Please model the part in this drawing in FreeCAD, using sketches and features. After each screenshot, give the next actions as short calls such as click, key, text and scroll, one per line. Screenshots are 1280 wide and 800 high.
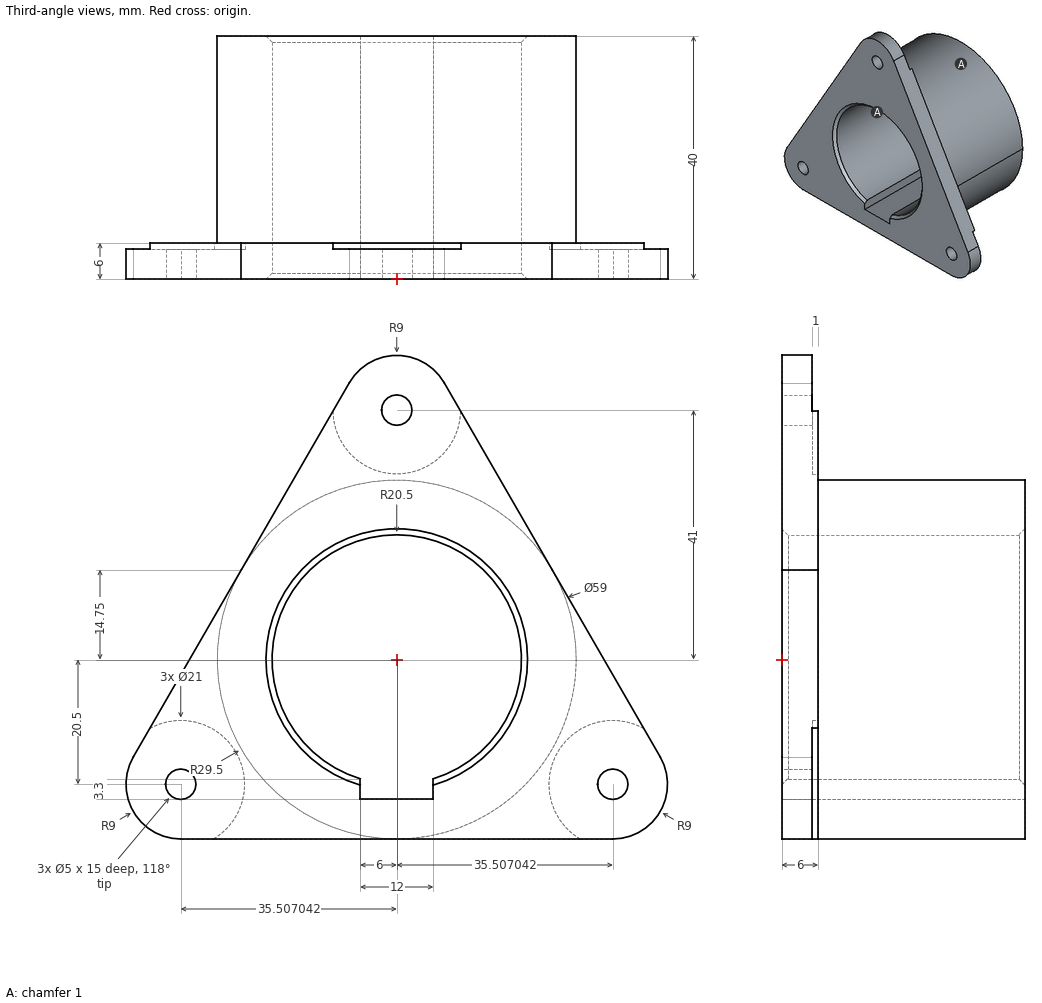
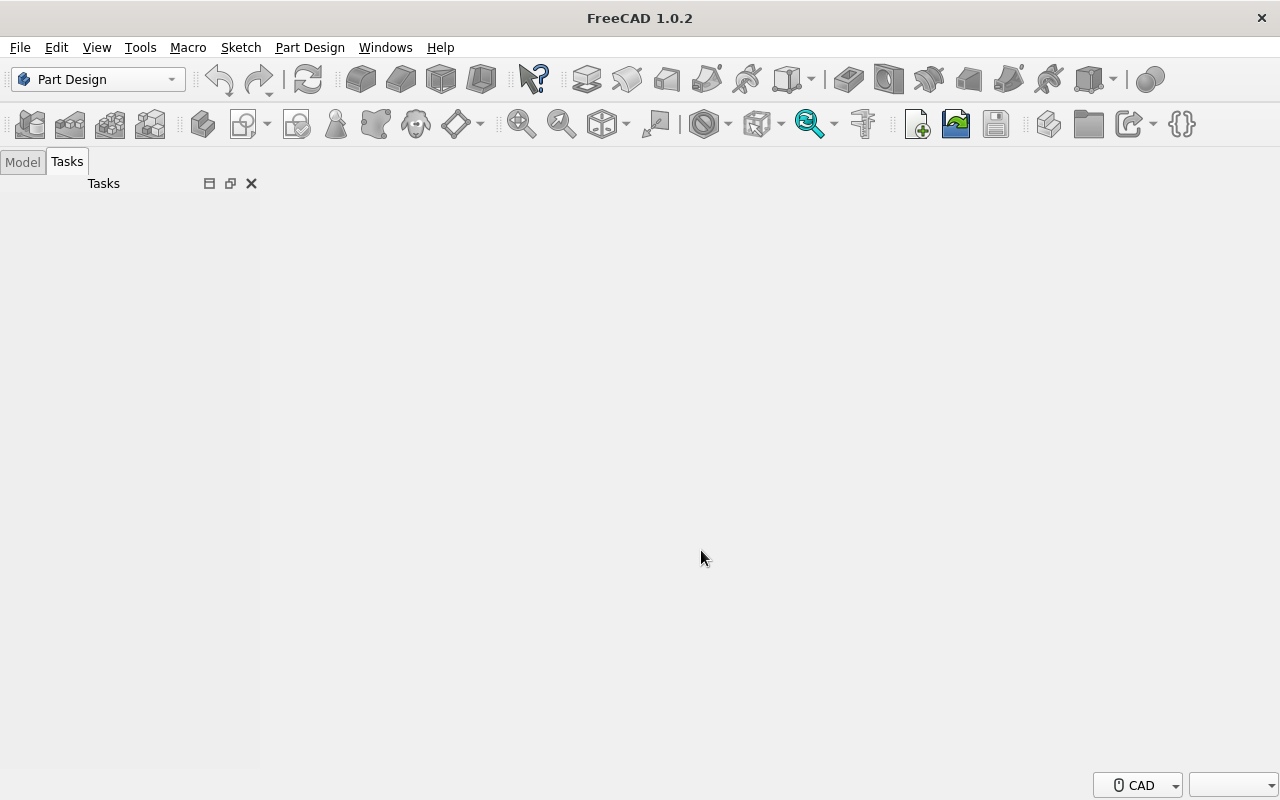
click(916, 124)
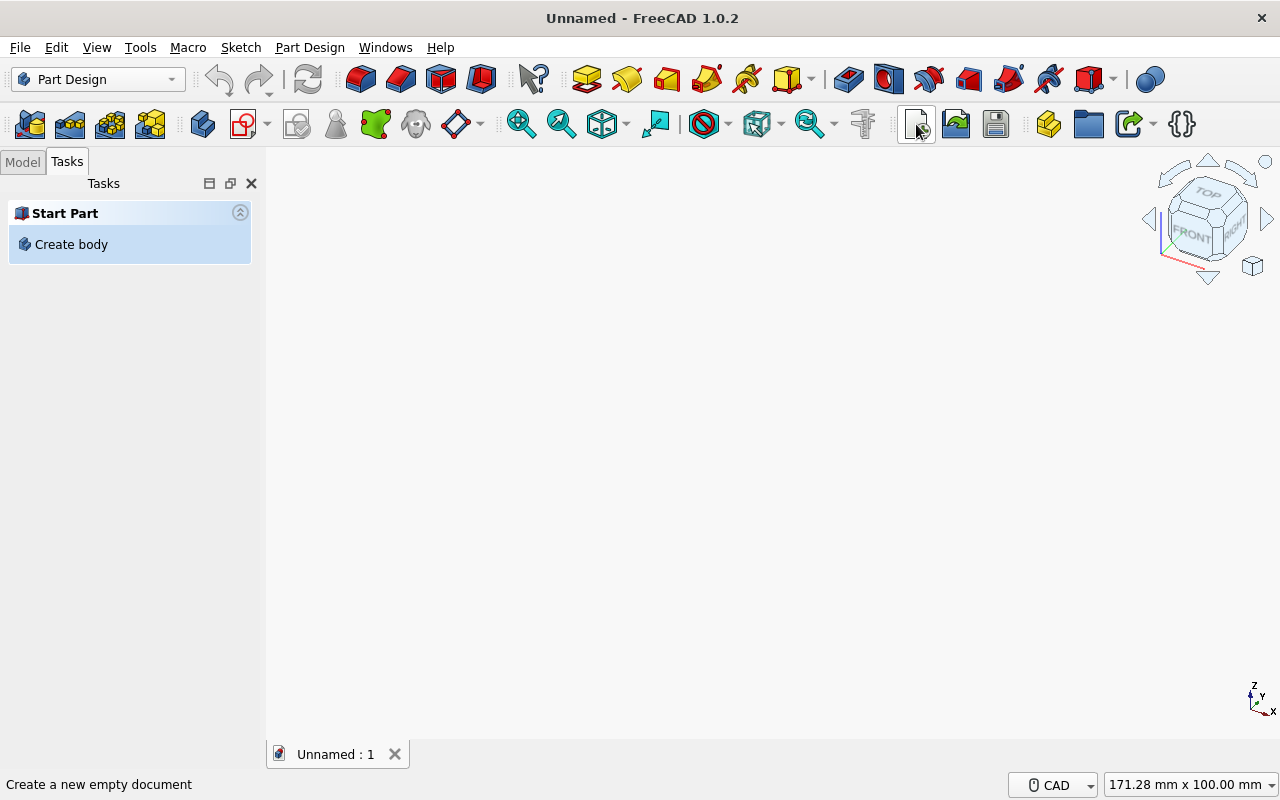
click(244, 124)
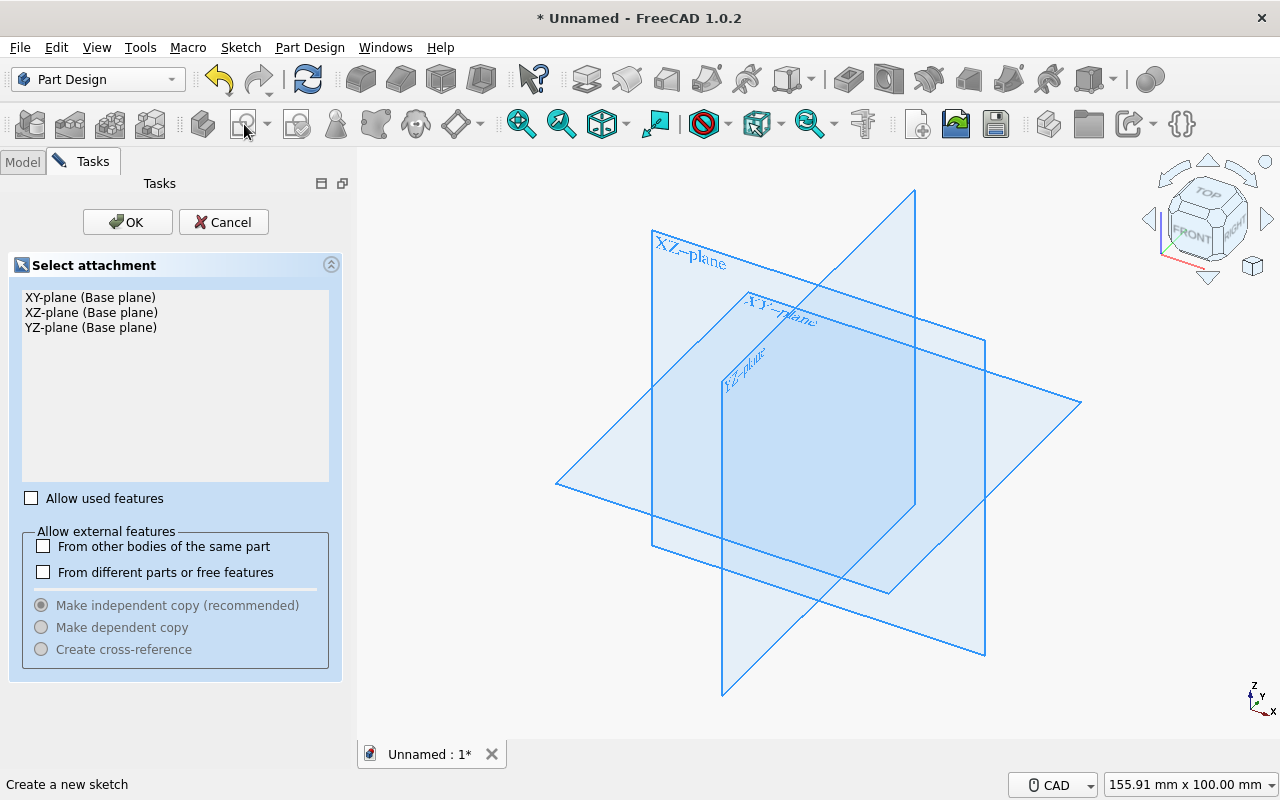
click(82, 312)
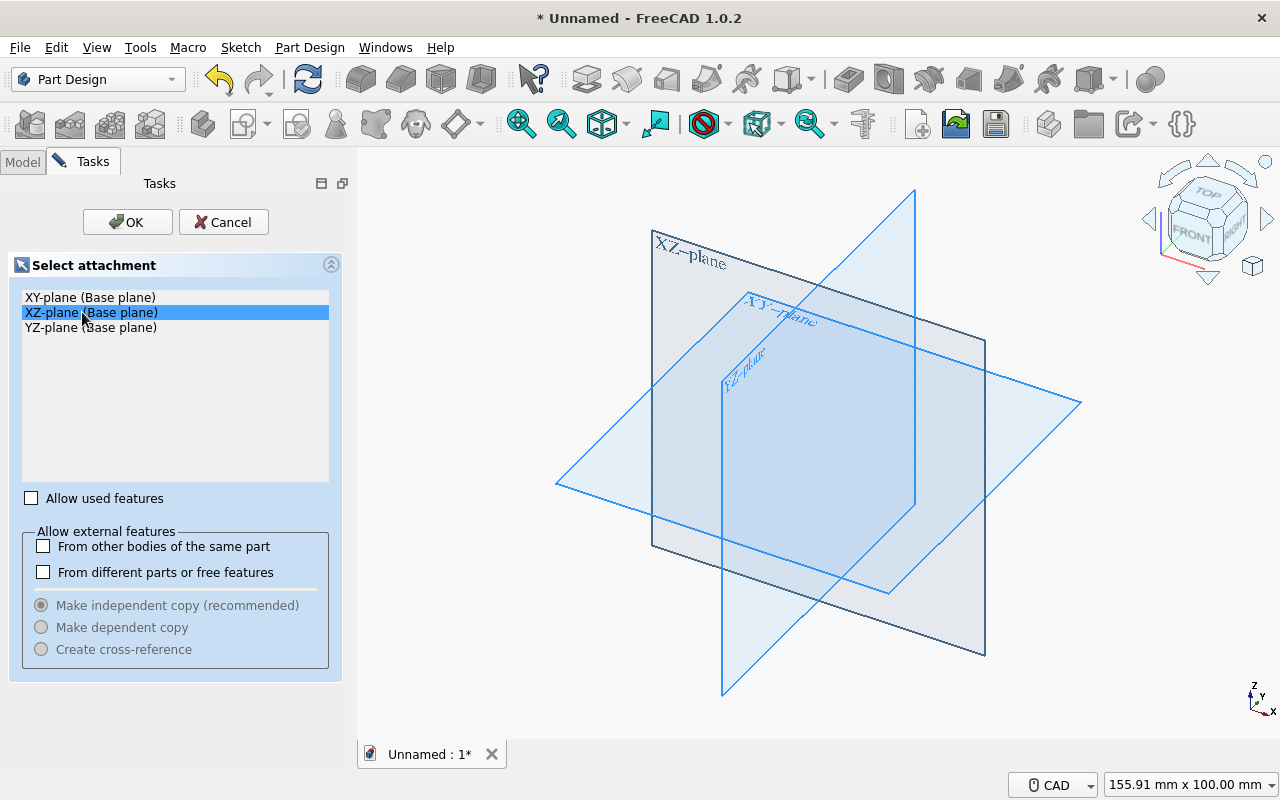
click(128, 222)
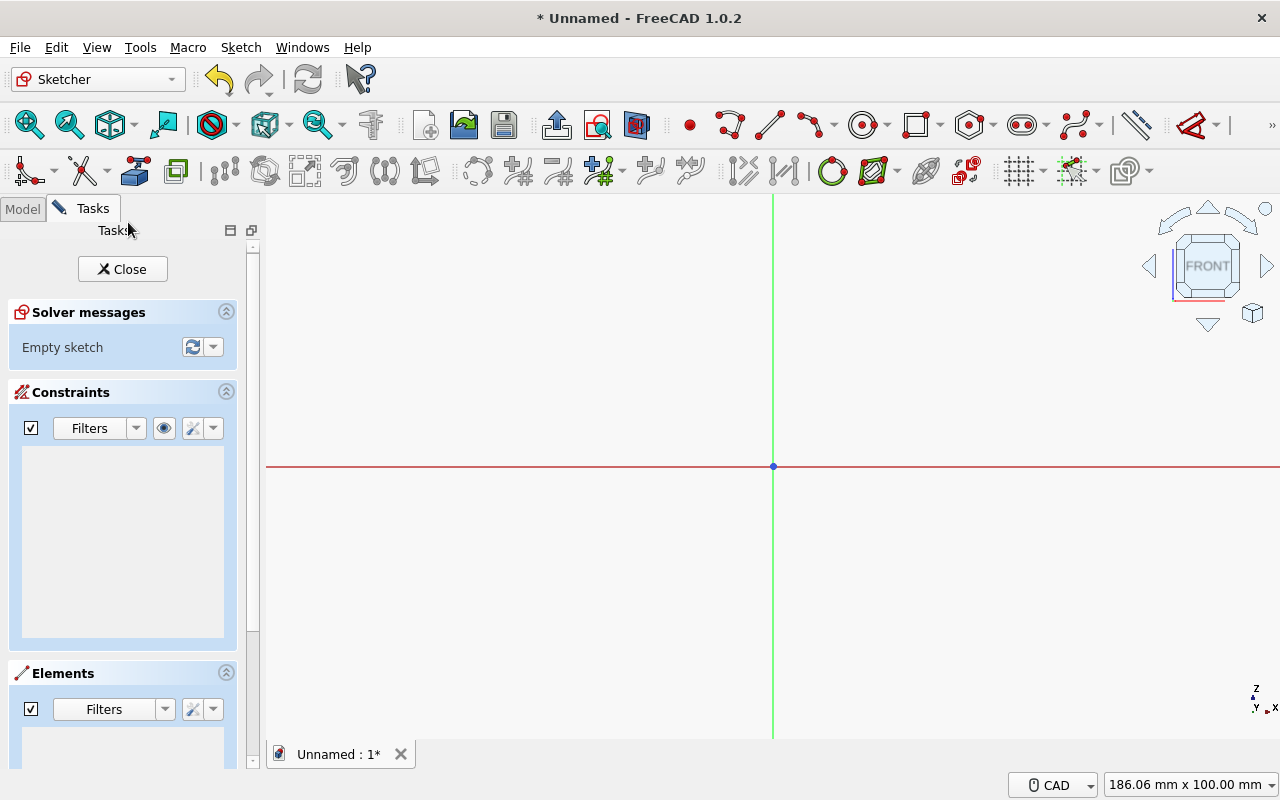
scroll(554, 588, up, 2)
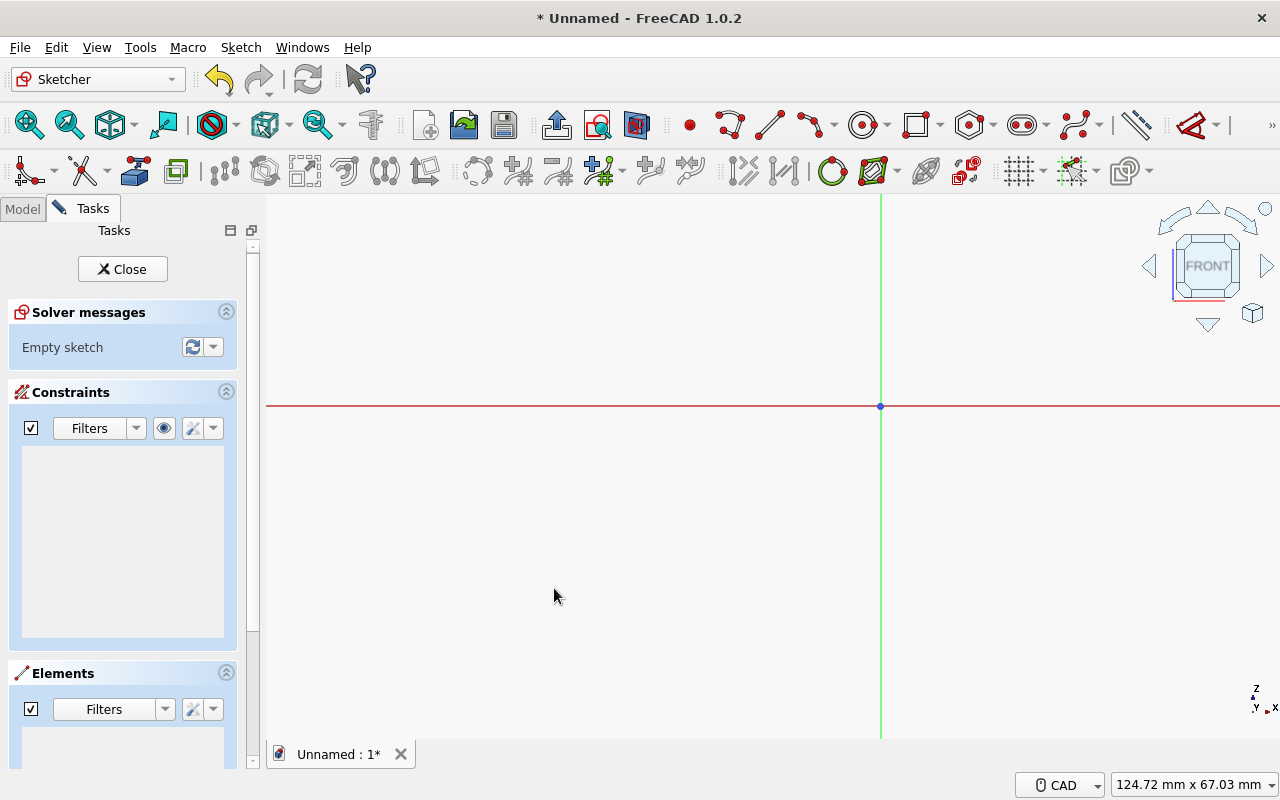
click(770, 126)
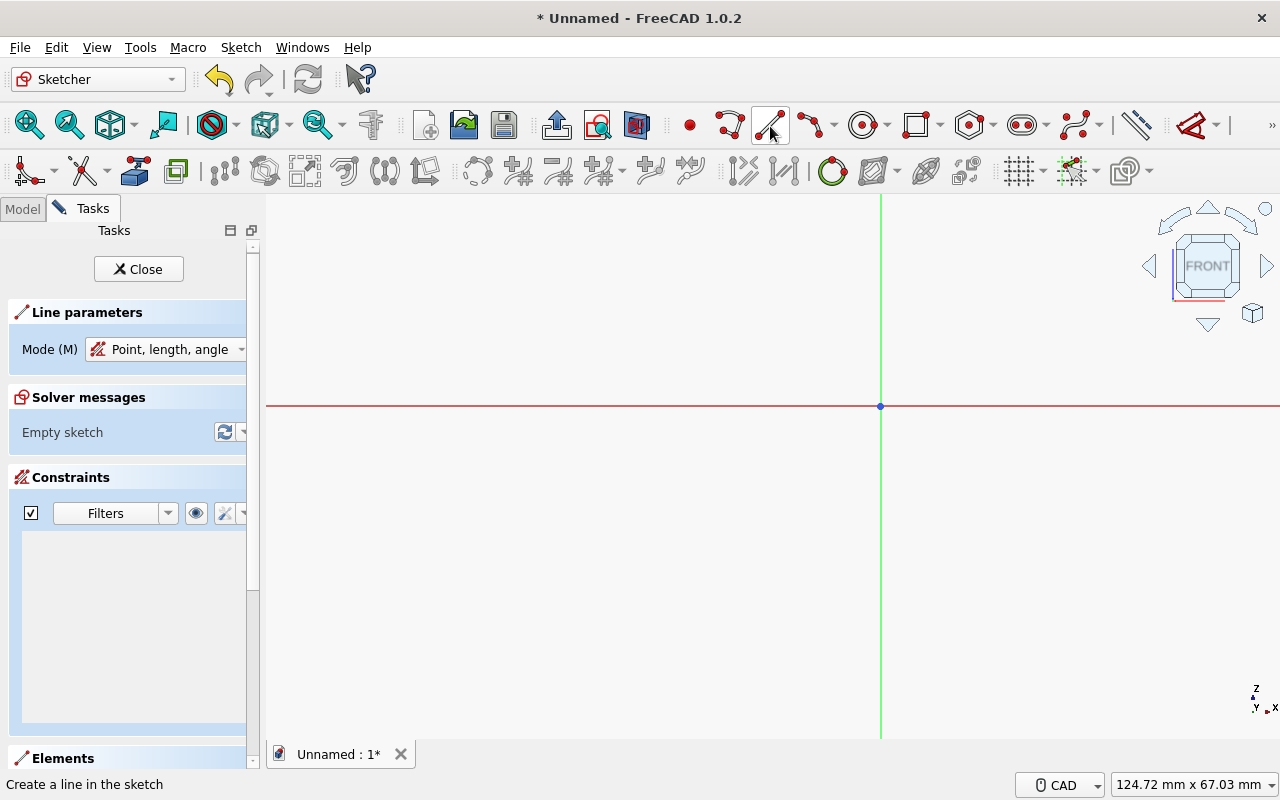
click(881, 646)
click(592, 646)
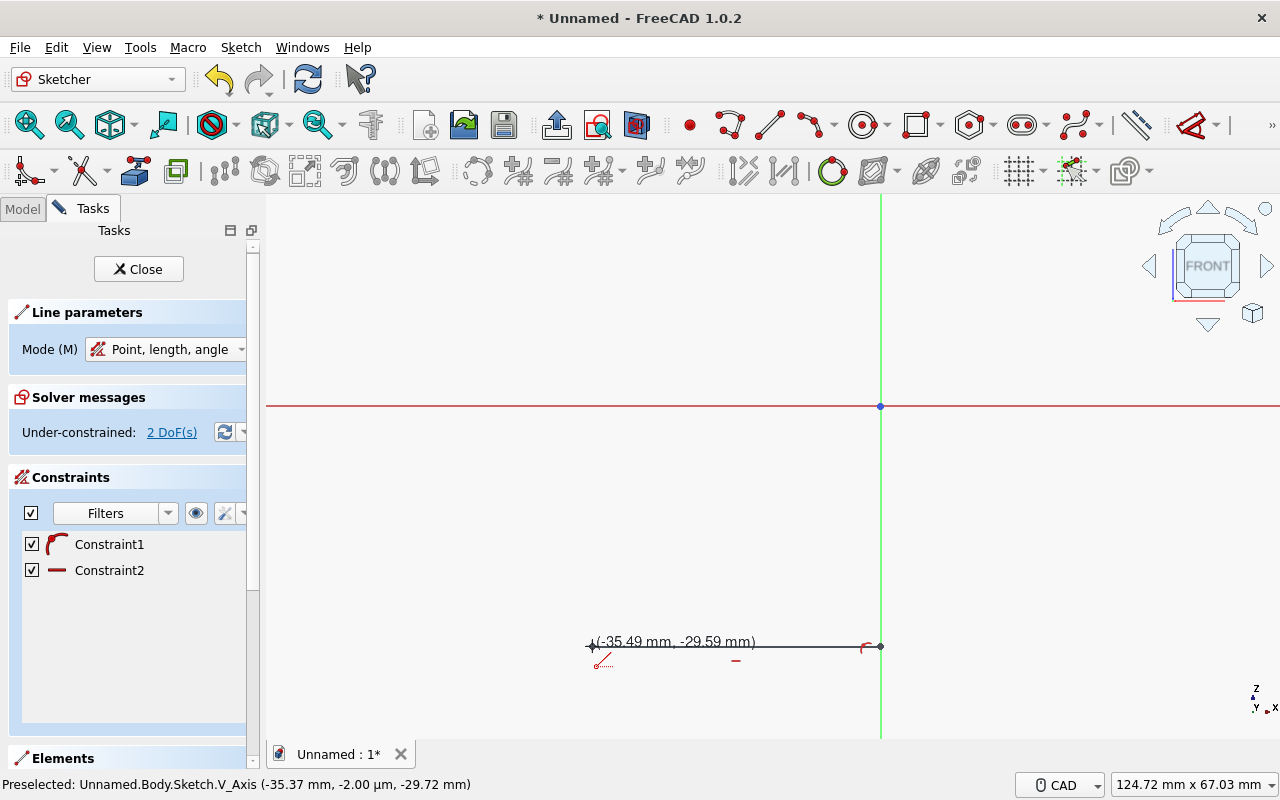
click(529, 536)
click(673, 286)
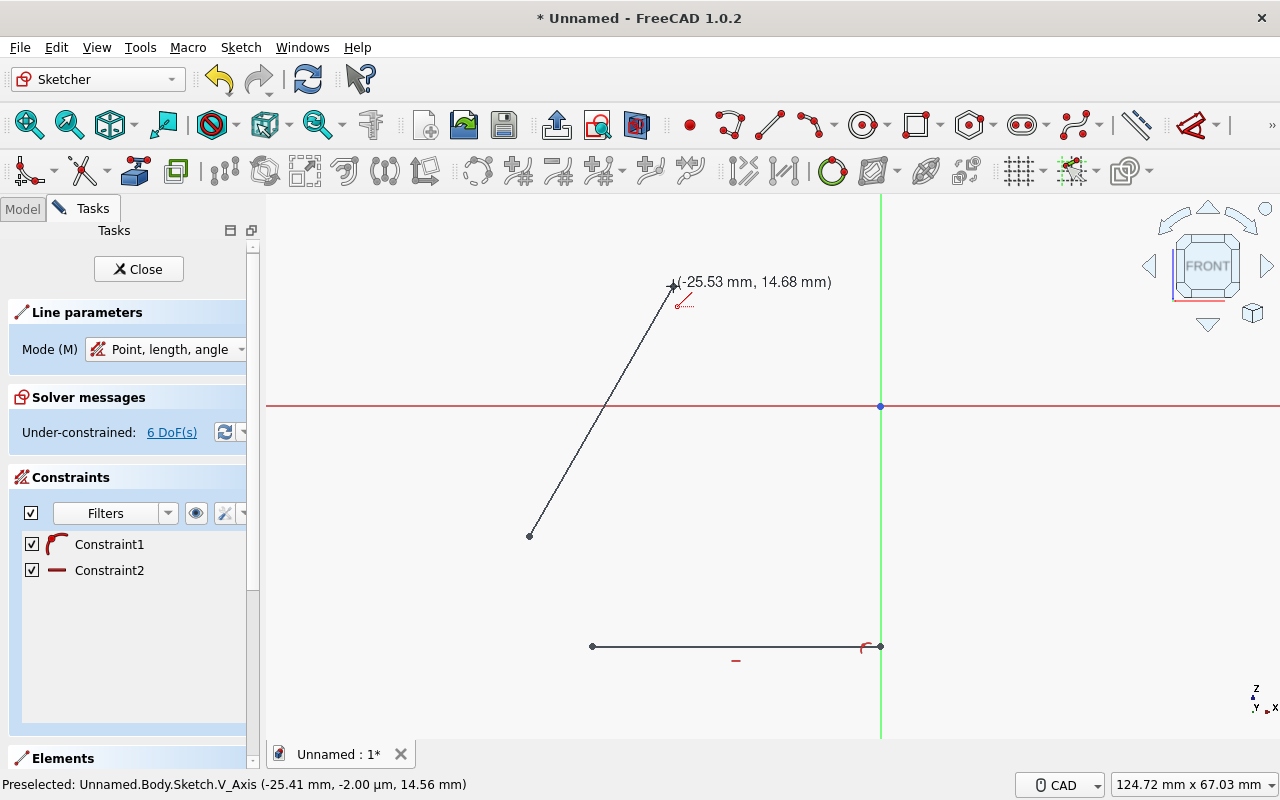
click(810, 126)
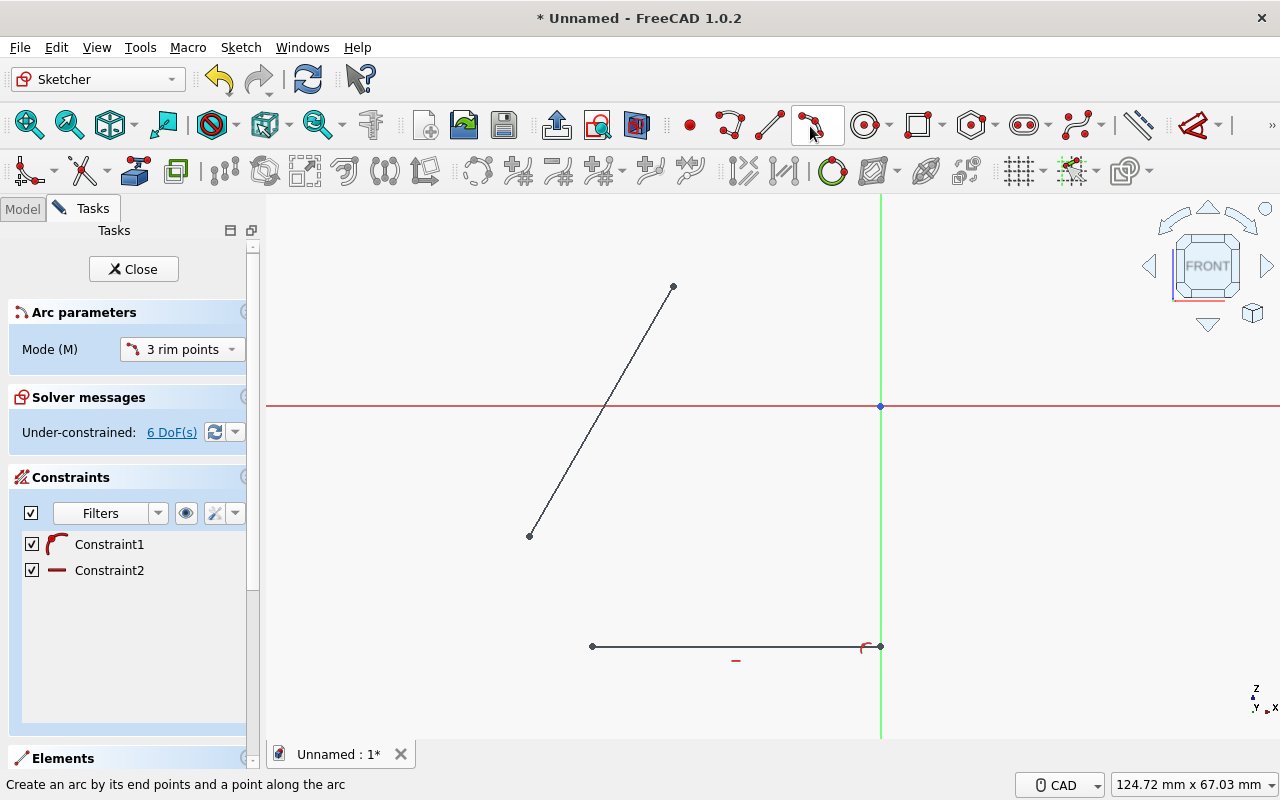
click(592, 647)
click(529, 537)
click(529, 610)